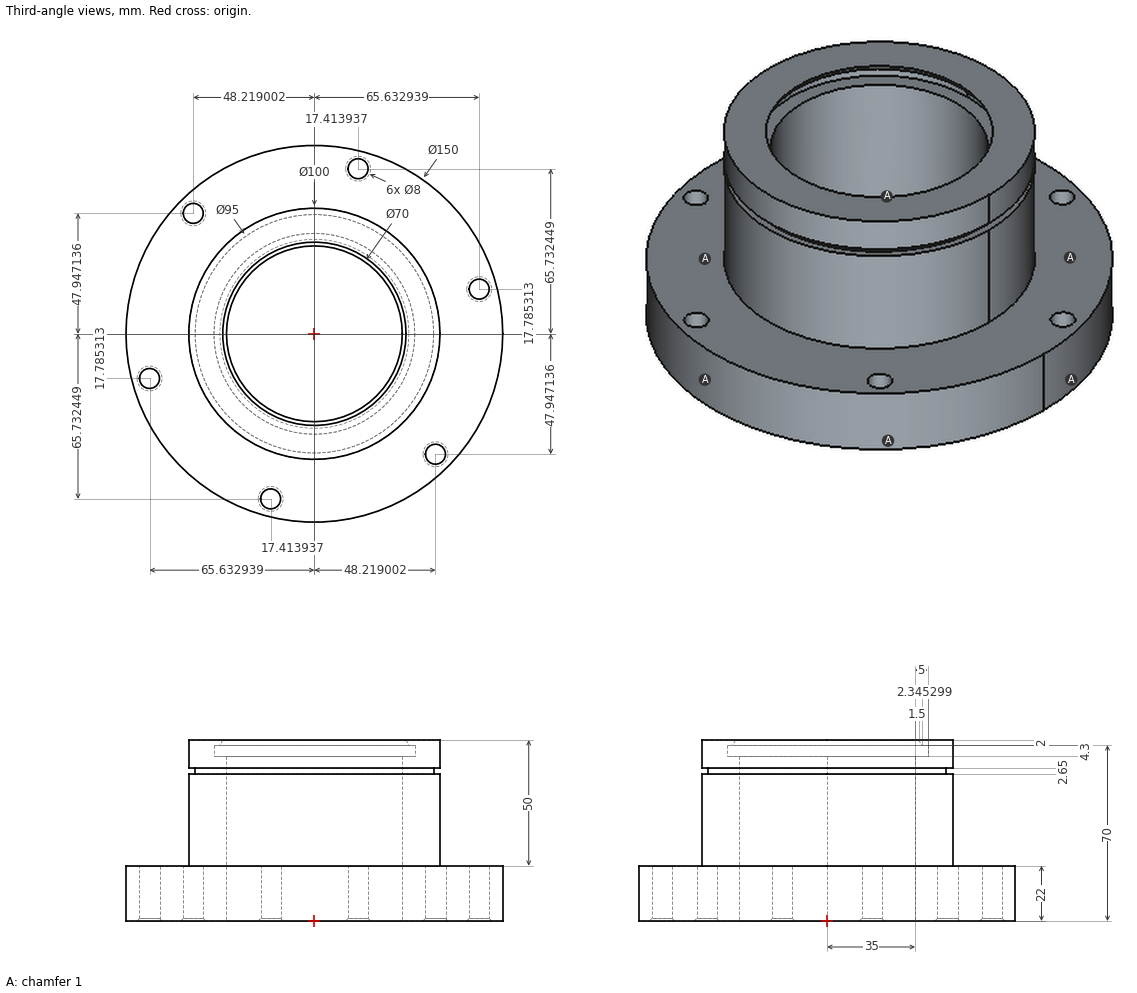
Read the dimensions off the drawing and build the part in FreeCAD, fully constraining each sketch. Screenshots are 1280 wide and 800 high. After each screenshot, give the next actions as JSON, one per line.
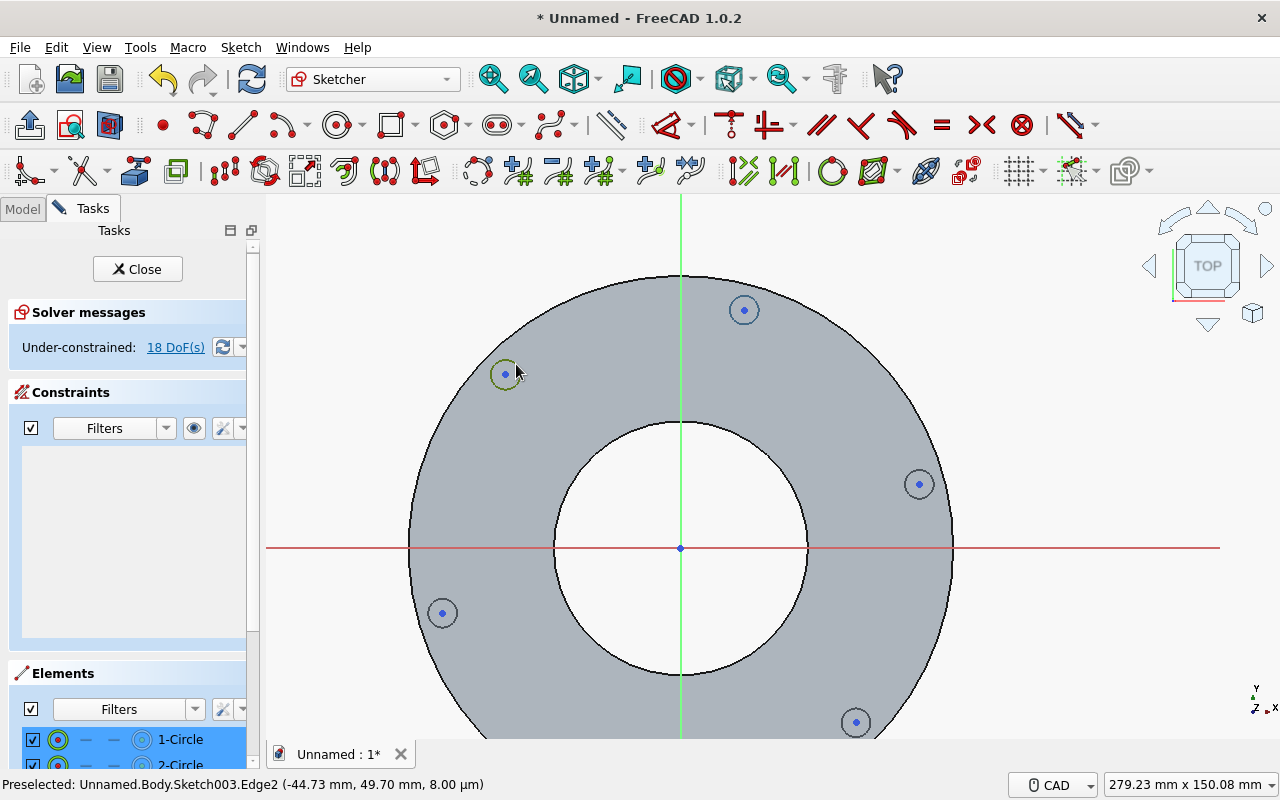
{"action": "left_click", "coordinate": [453, 603]}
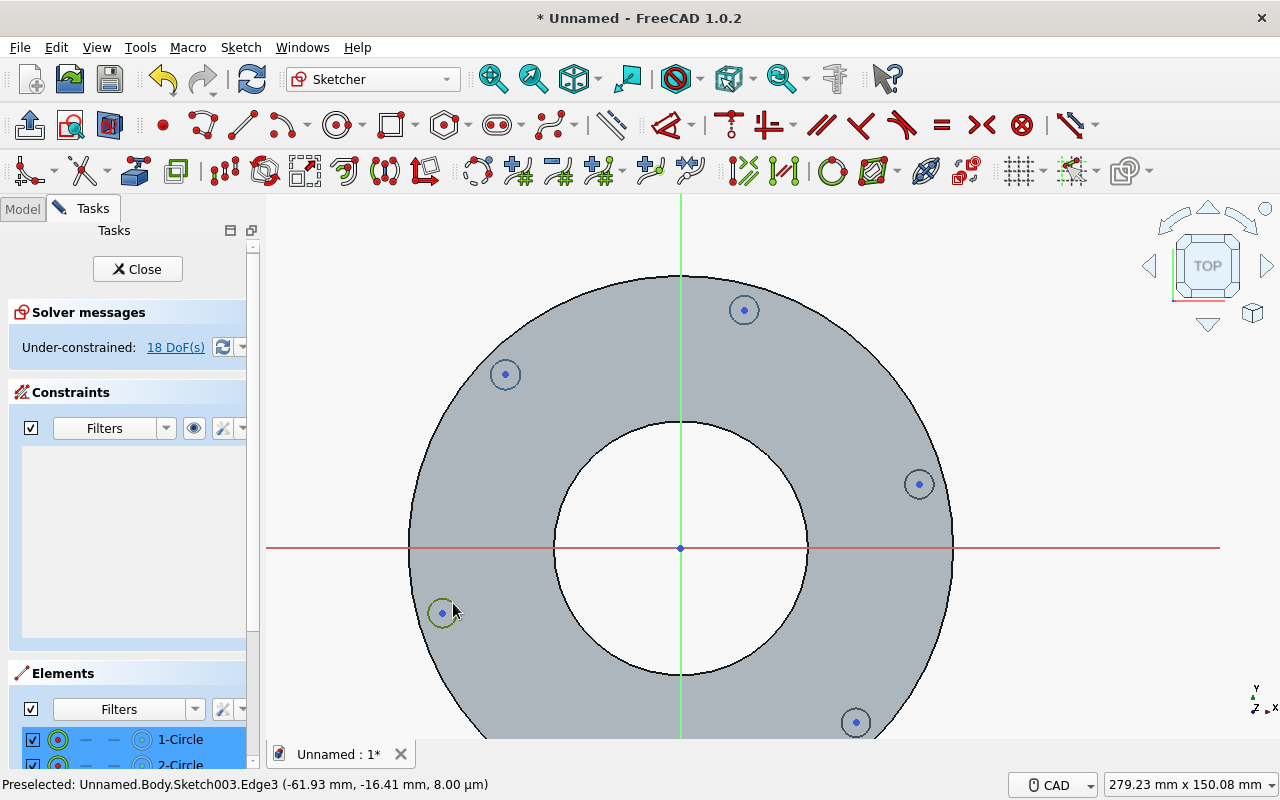
{"action": "scroll", "coordinate": [753, 300], "scroll_direction": "down", "scroll_amount": 2}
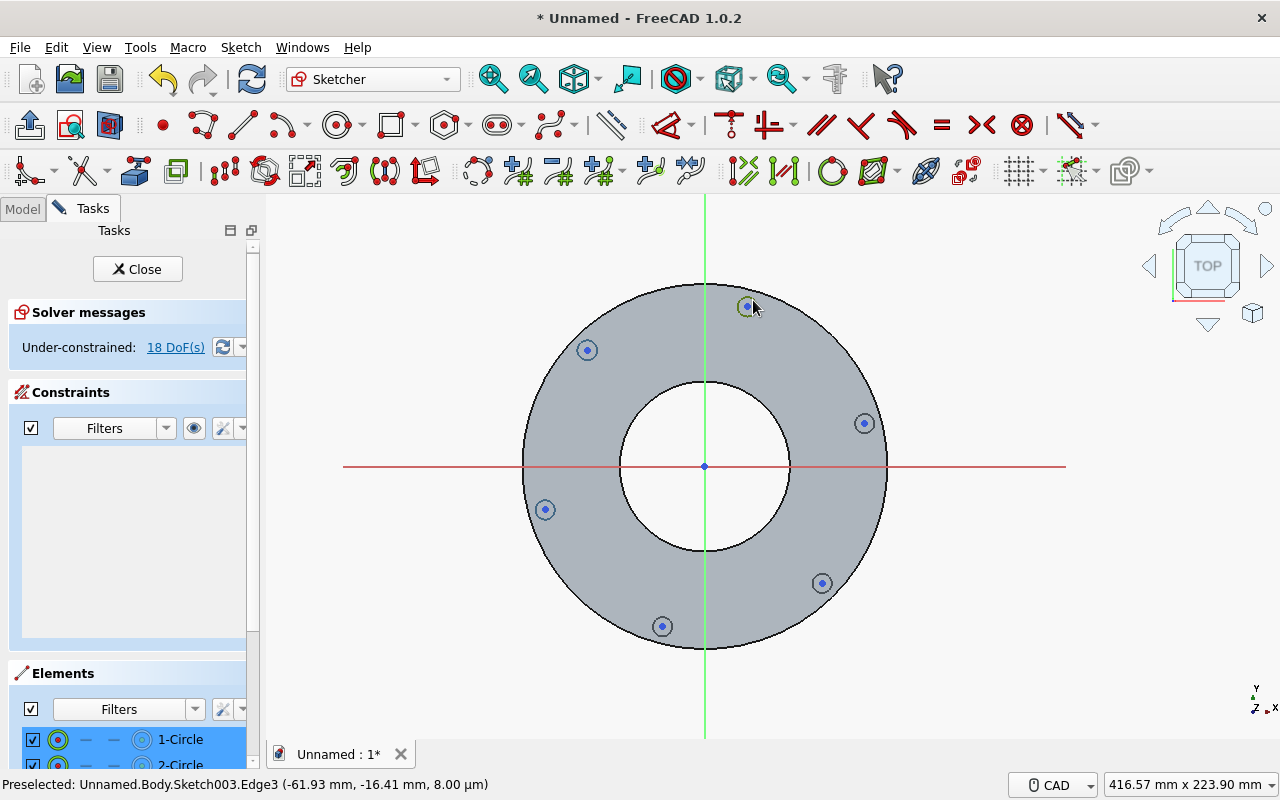
{"action": "scroll", "coordinate": [669, 620], "scroll_direction": "up", "scroll_amount": 2}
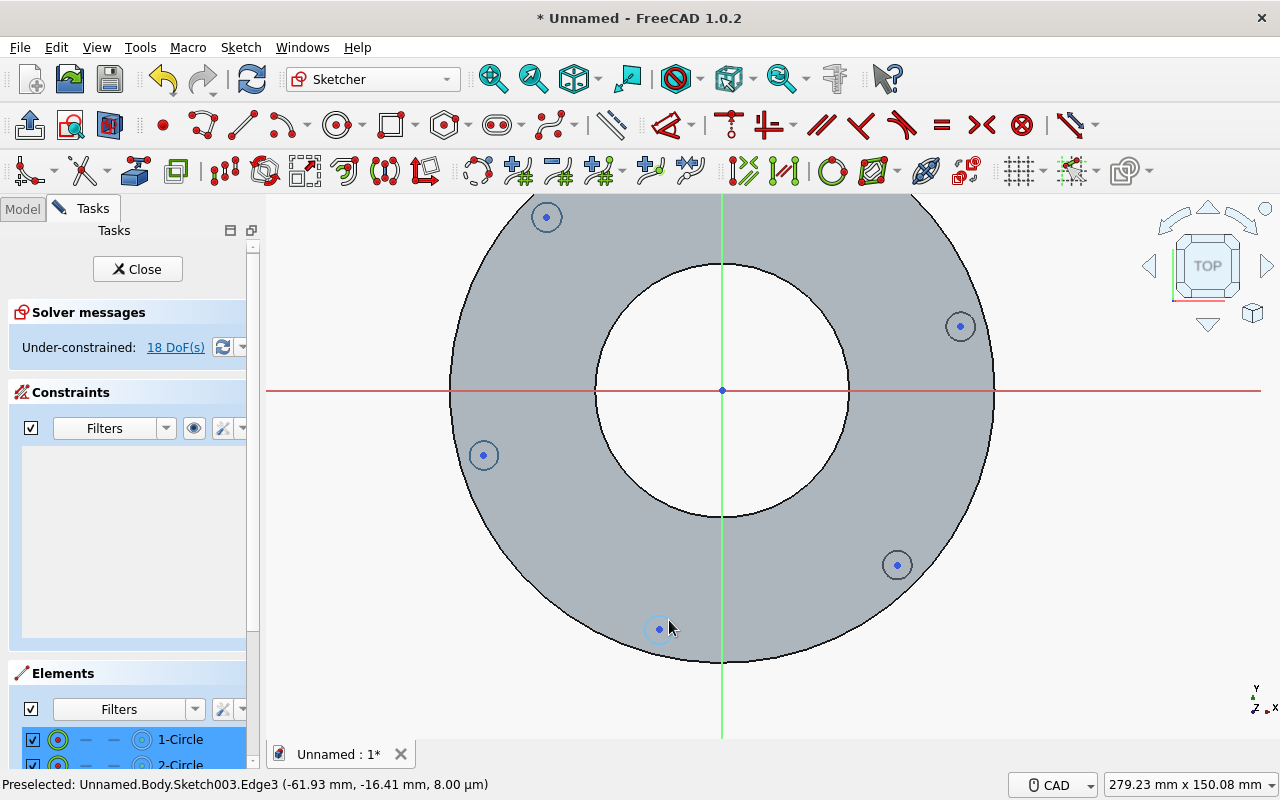
{"action": "left_click", "coordinate": [669, 620]}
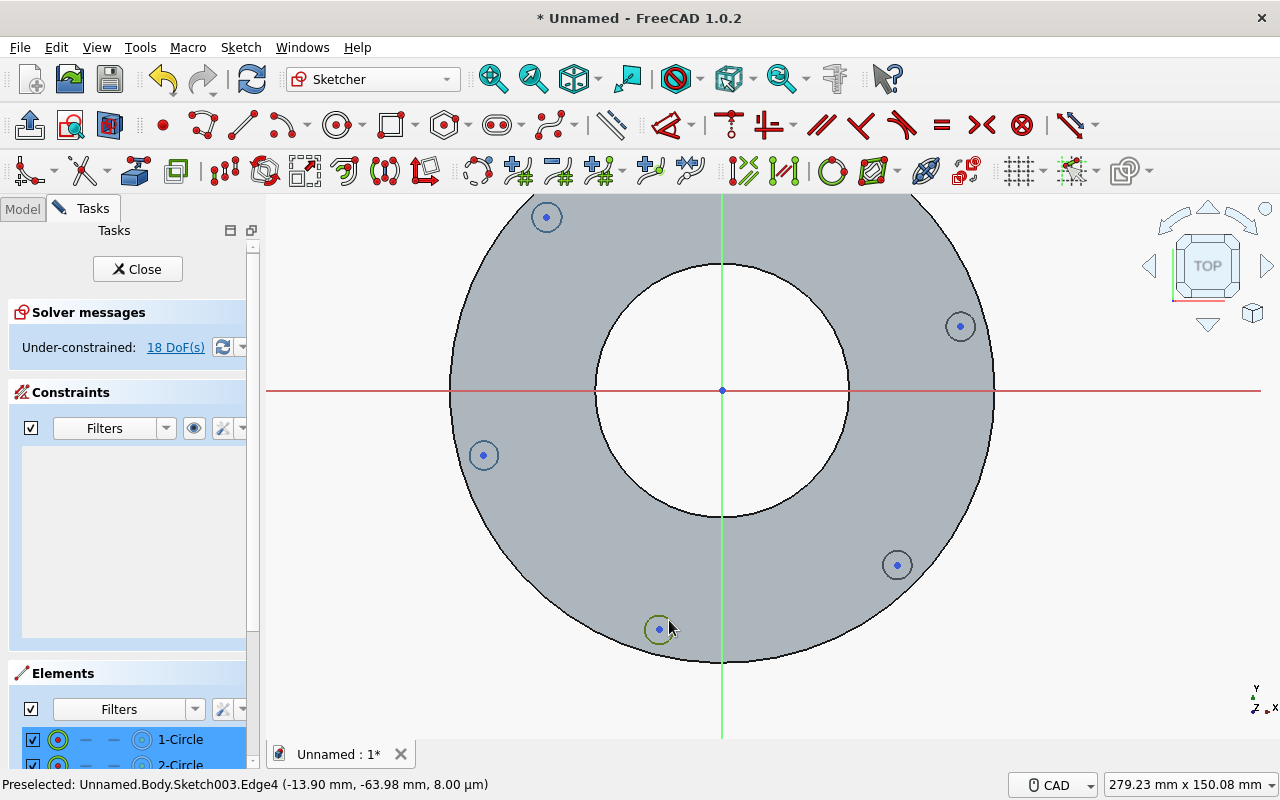
{"action": "left_click", "coordinate": [907, 555]}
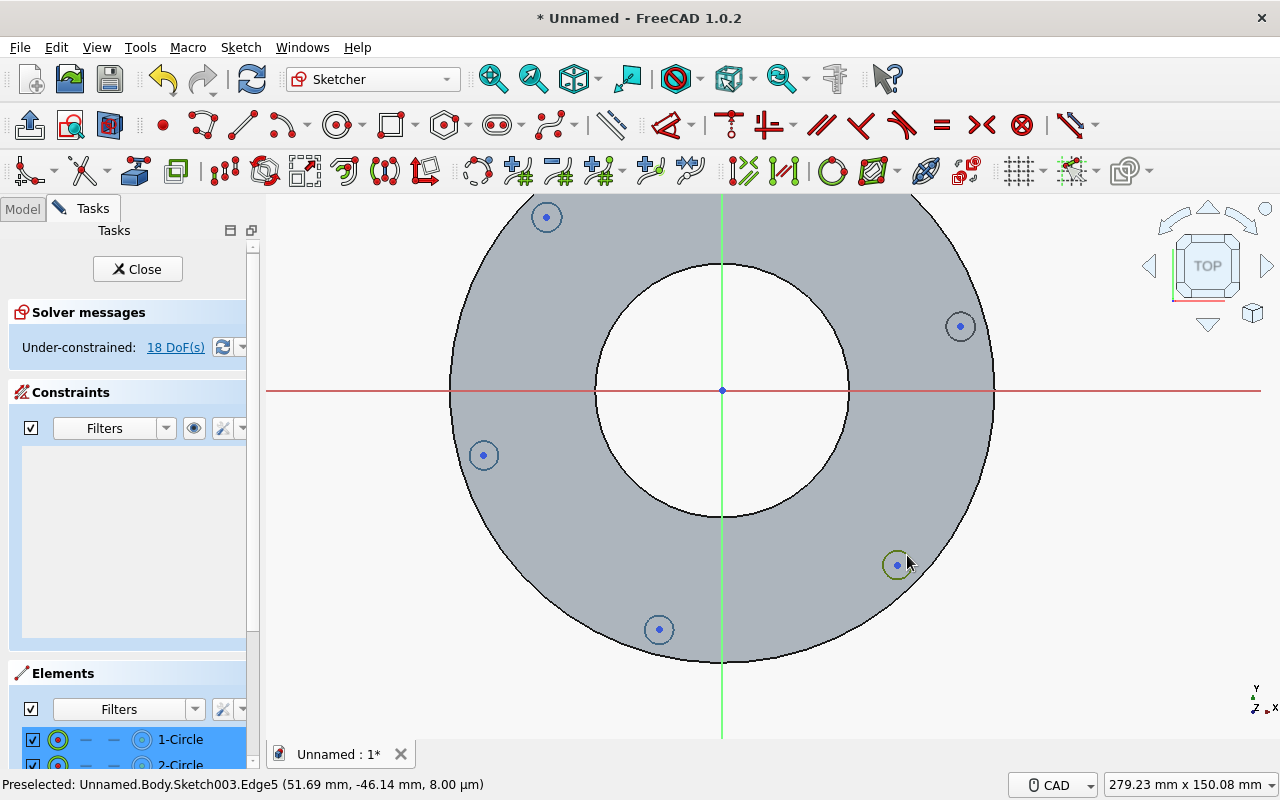
{"action": "left_click", "coordinate": [971, 316]}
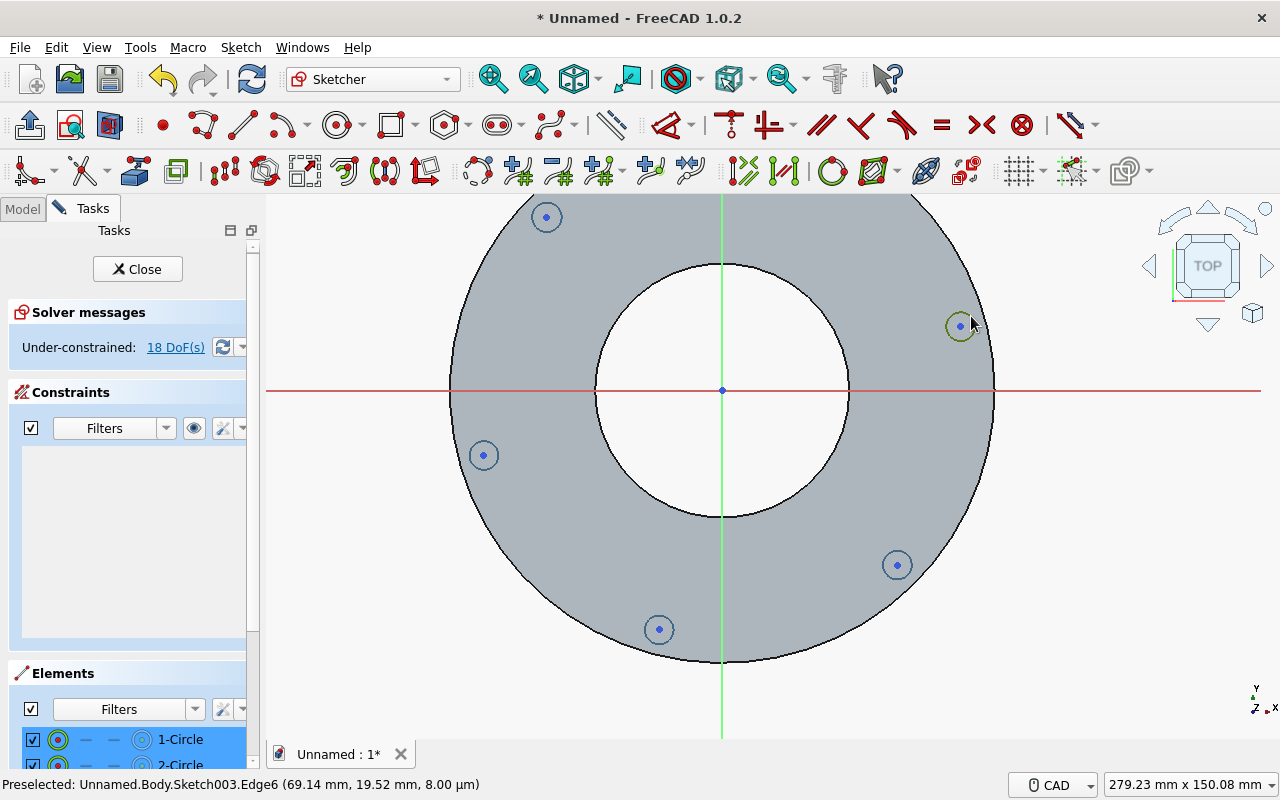
{"action": "left_click", "coordinate": [942, 126]}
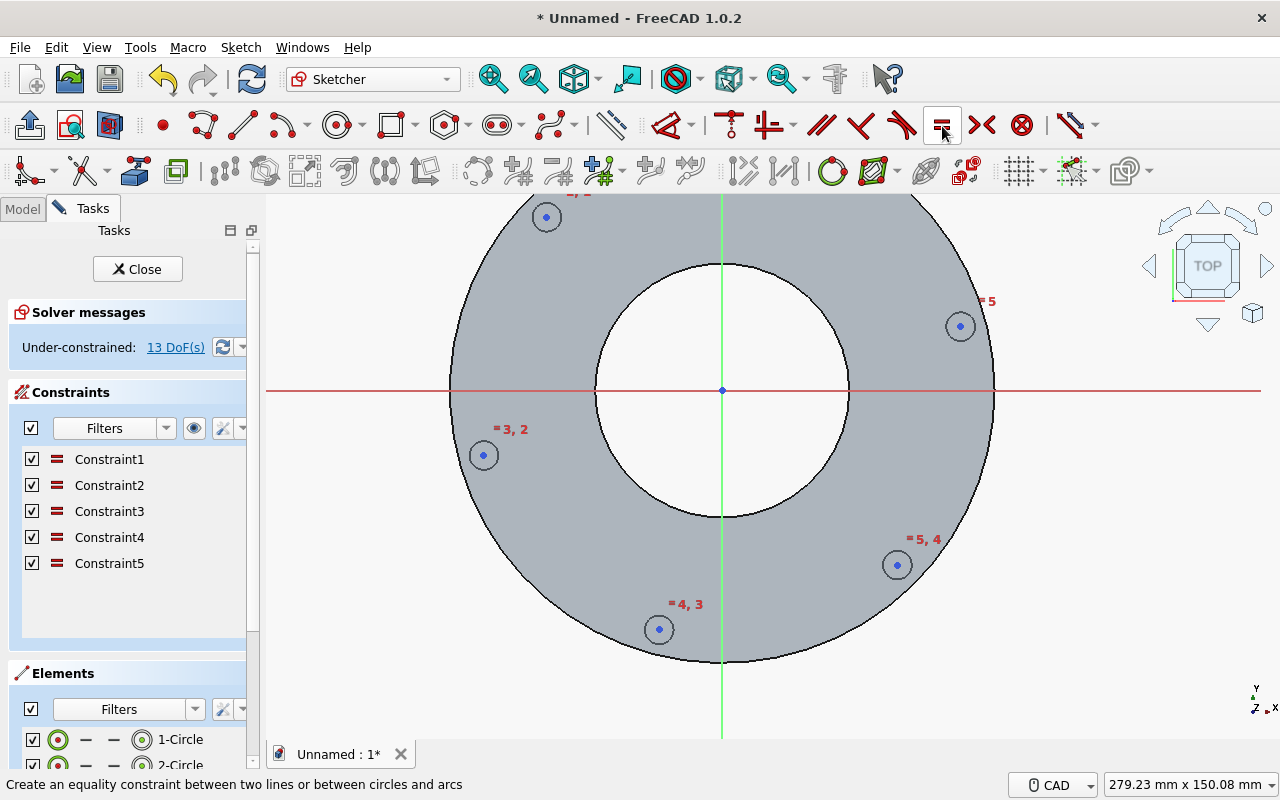
{"action": "key", "text": "d"}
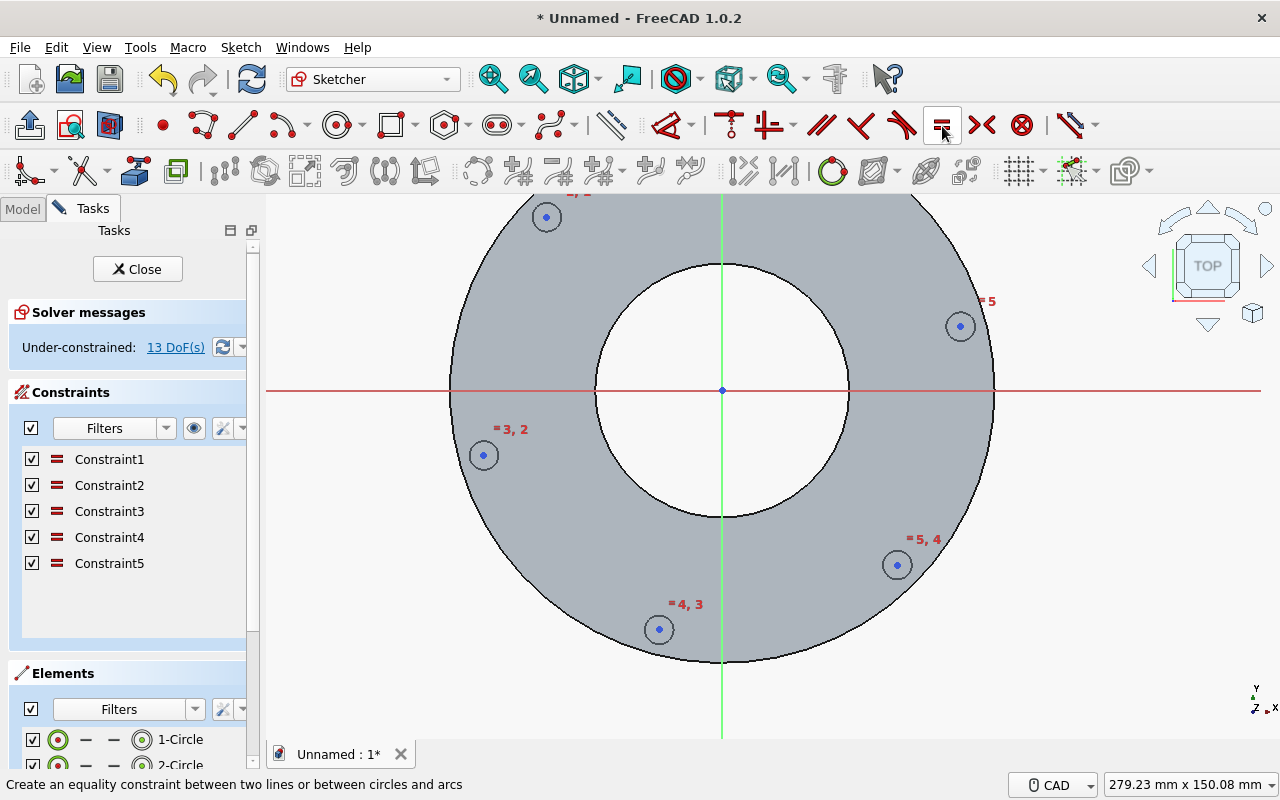
{"action": "scroll", "coordinate": [668, 621], "scroll_direction": "down", "scroll_amount": 2}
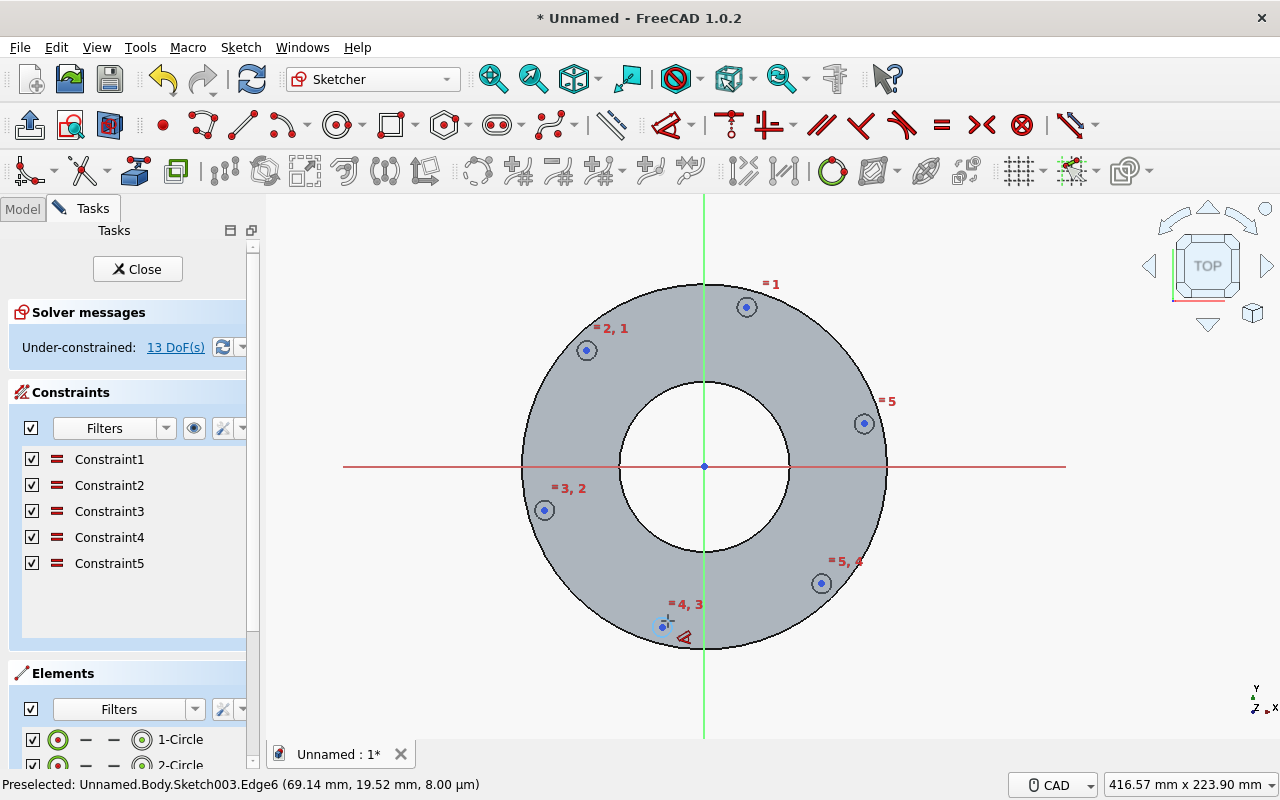
{"action": "scroll", "coordinate": [754, 300], "scroll_direction": "up", "scroll_amount": 4}